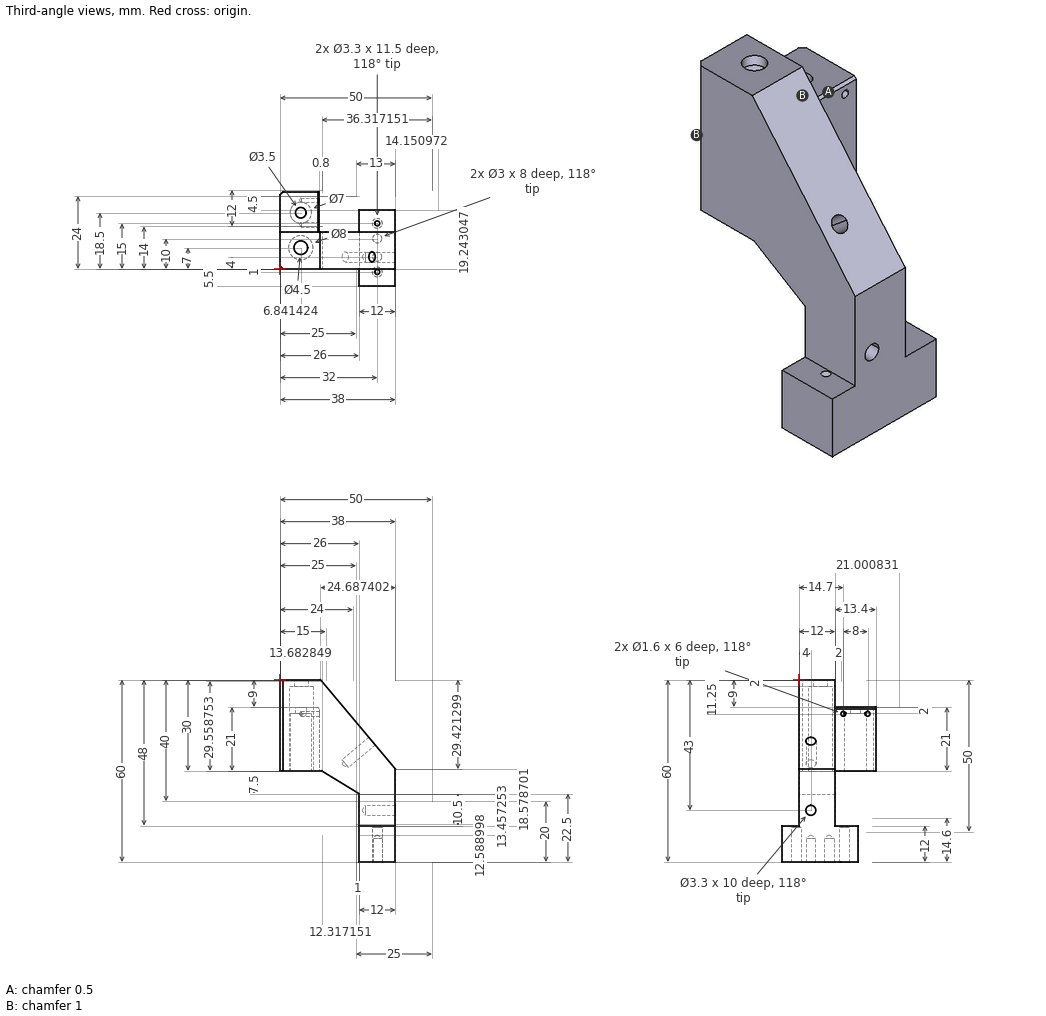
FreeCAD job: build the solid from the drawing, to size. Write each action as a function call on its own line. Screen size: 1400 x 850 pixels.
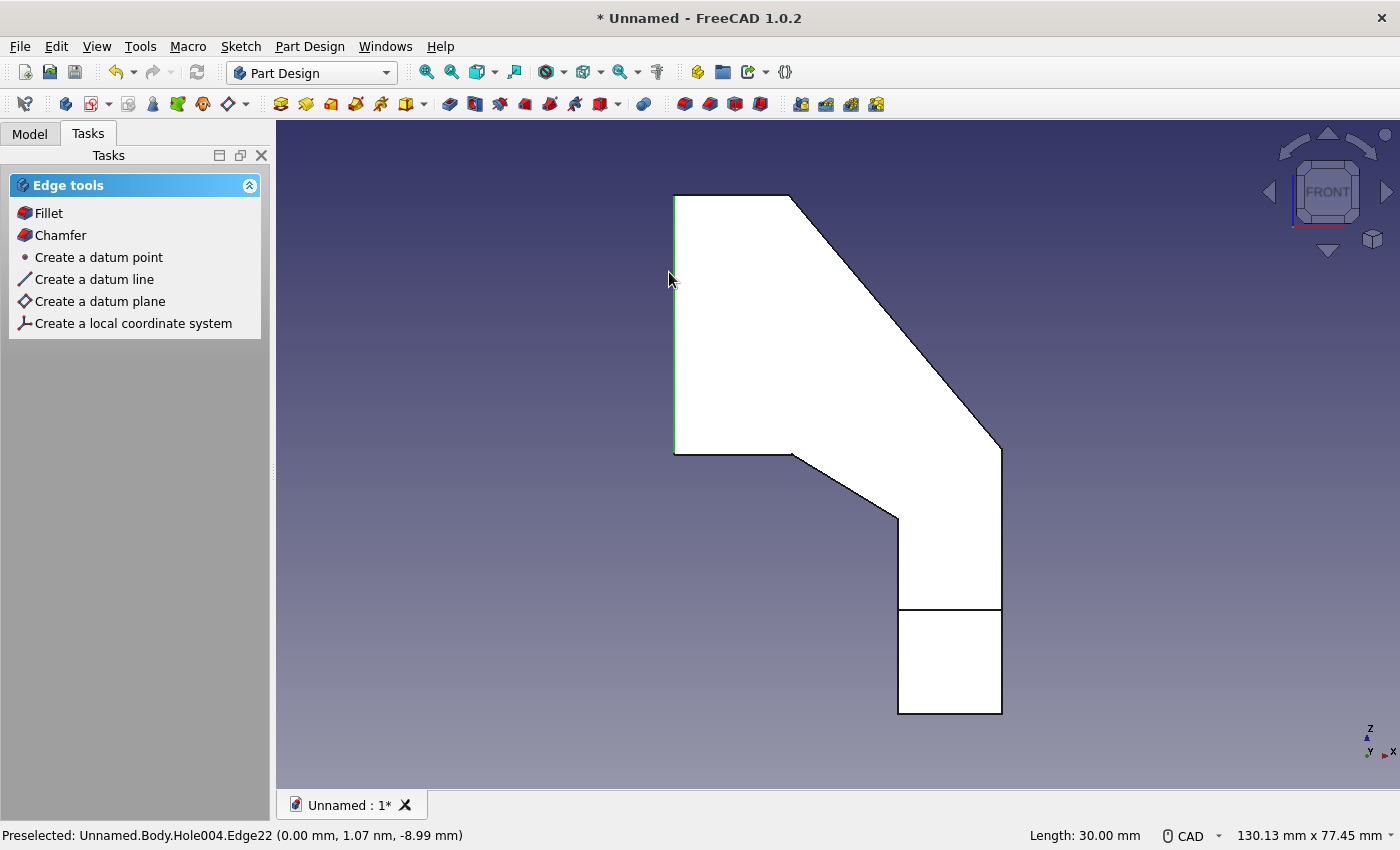
key(3)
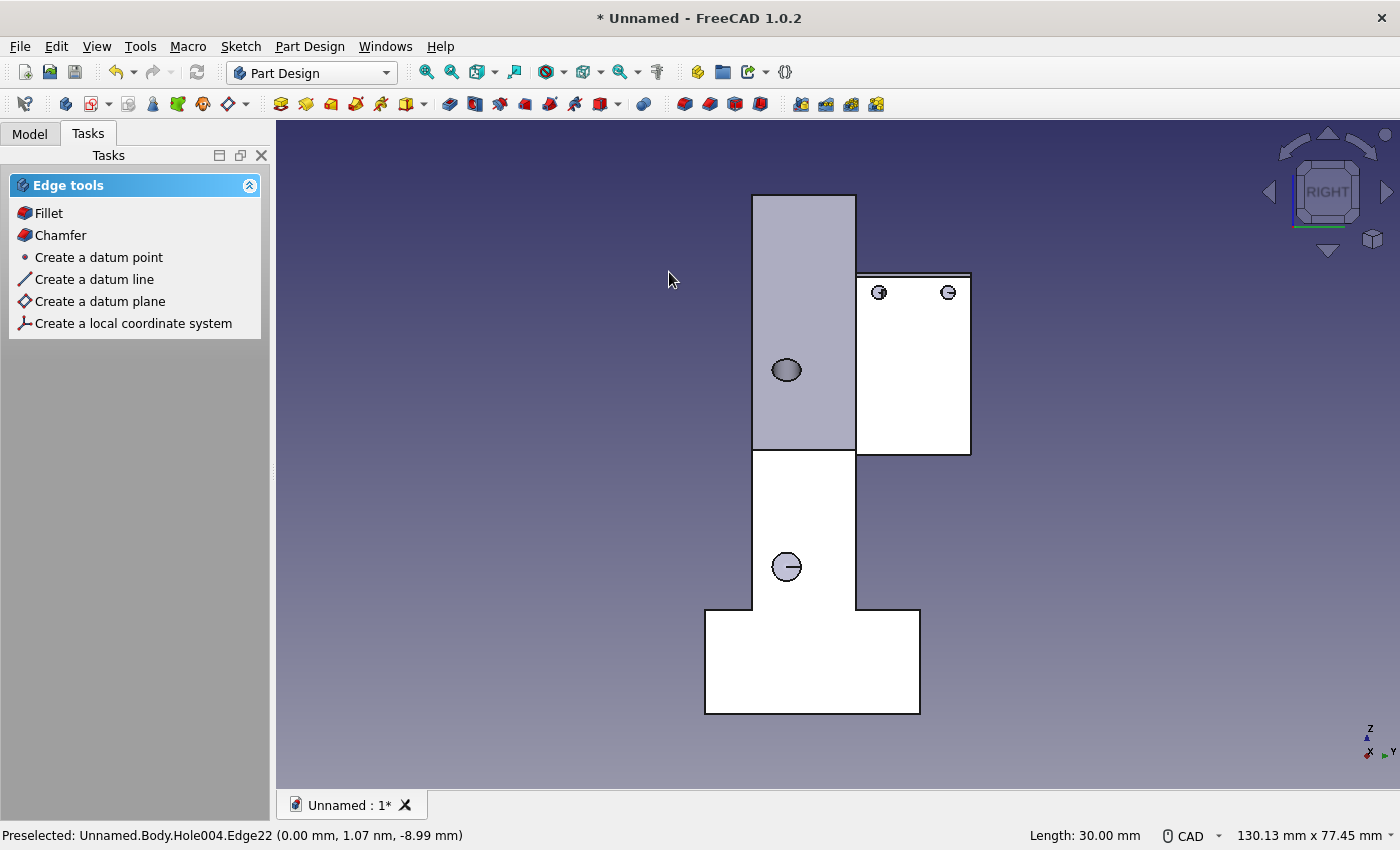
key(5)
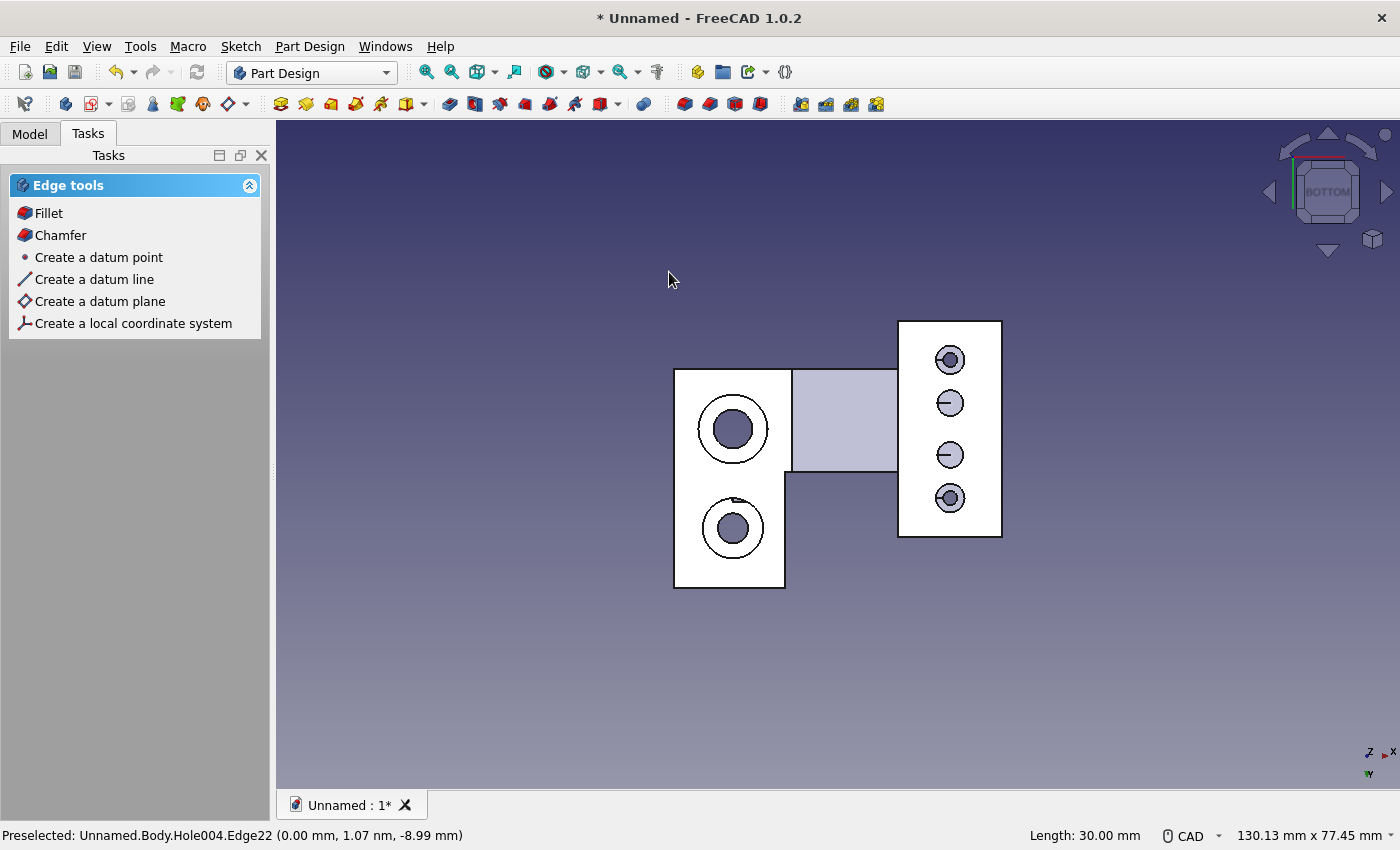
click(427, 72)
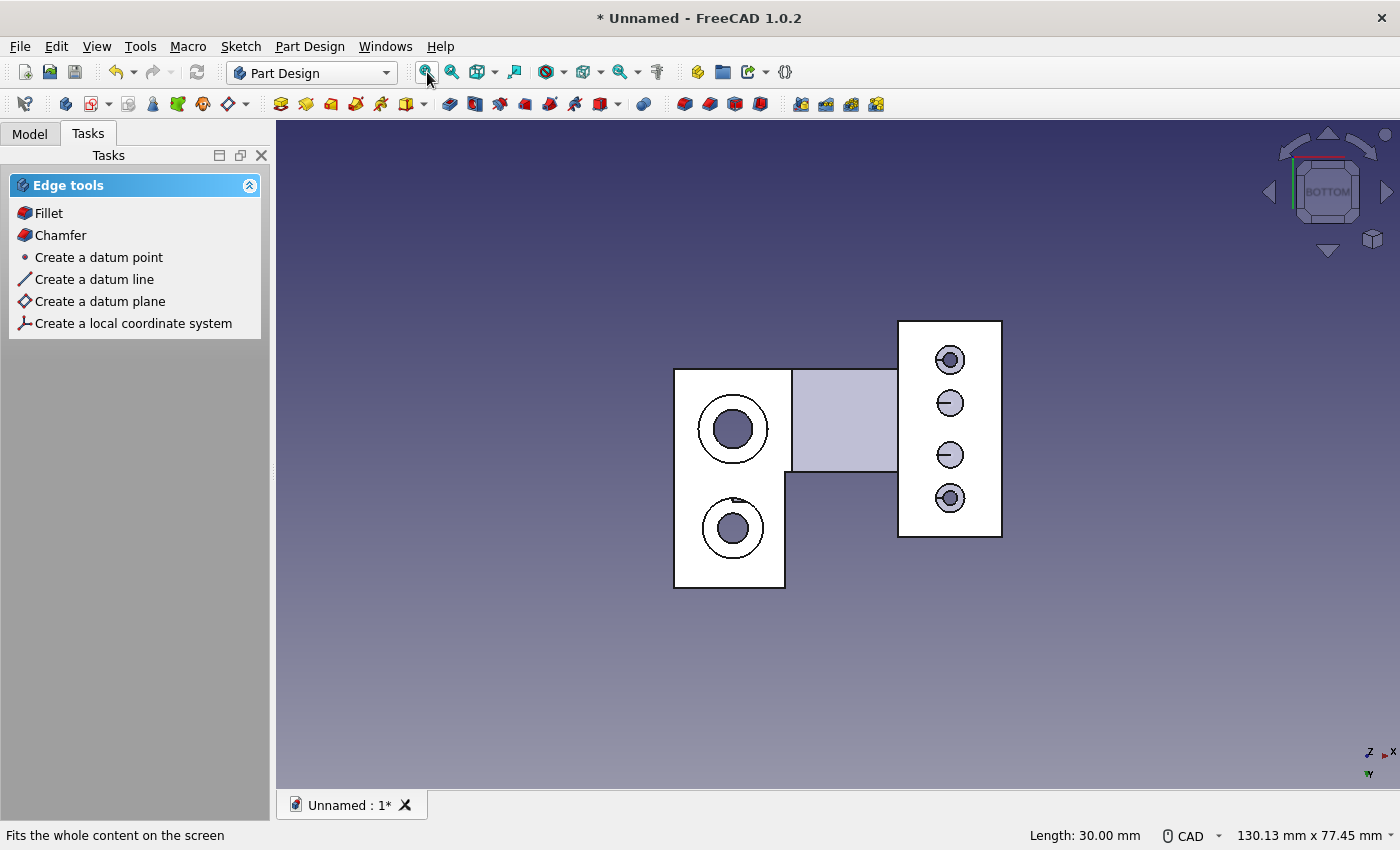
key(4)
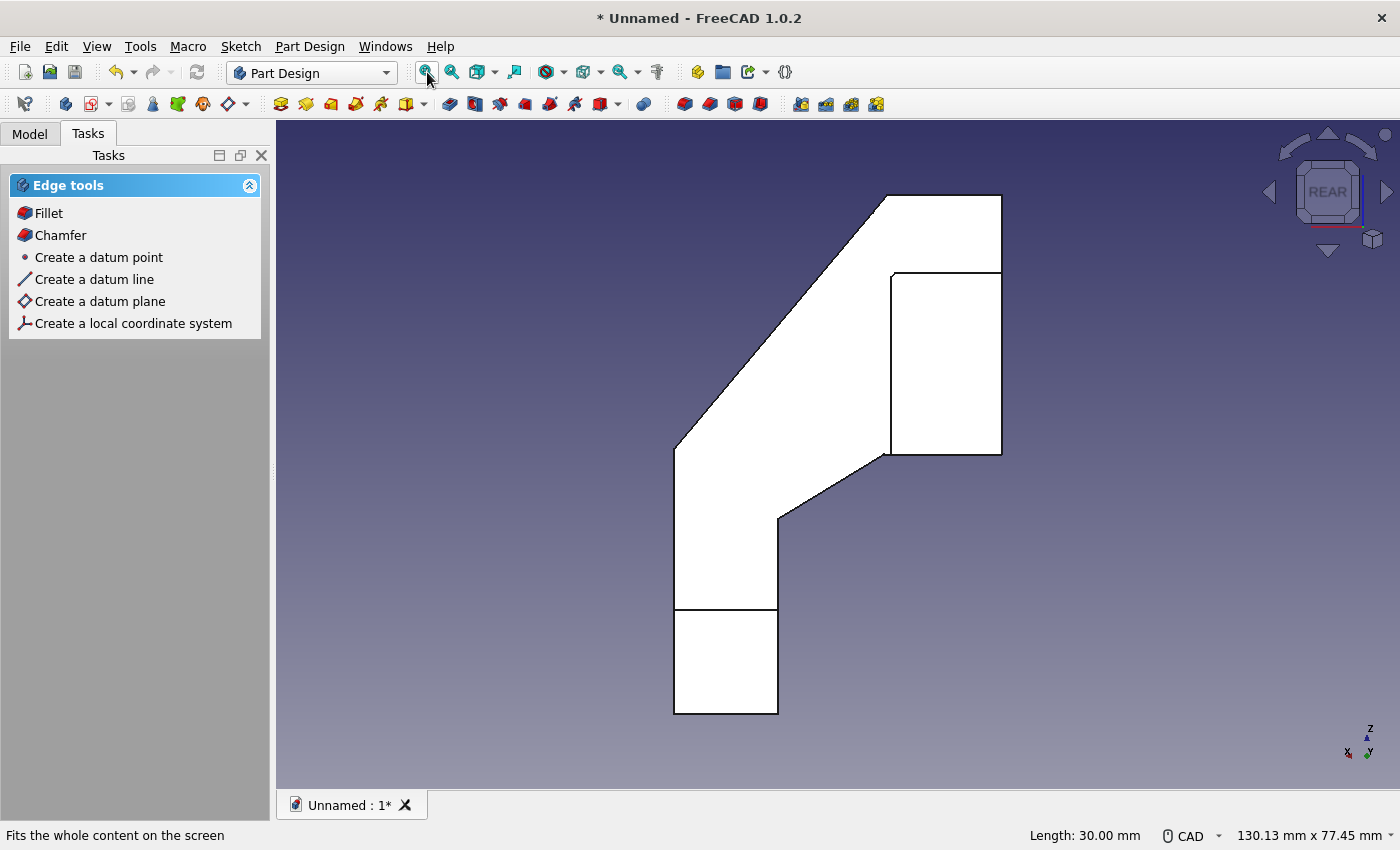
click(1002, 363, ctrl)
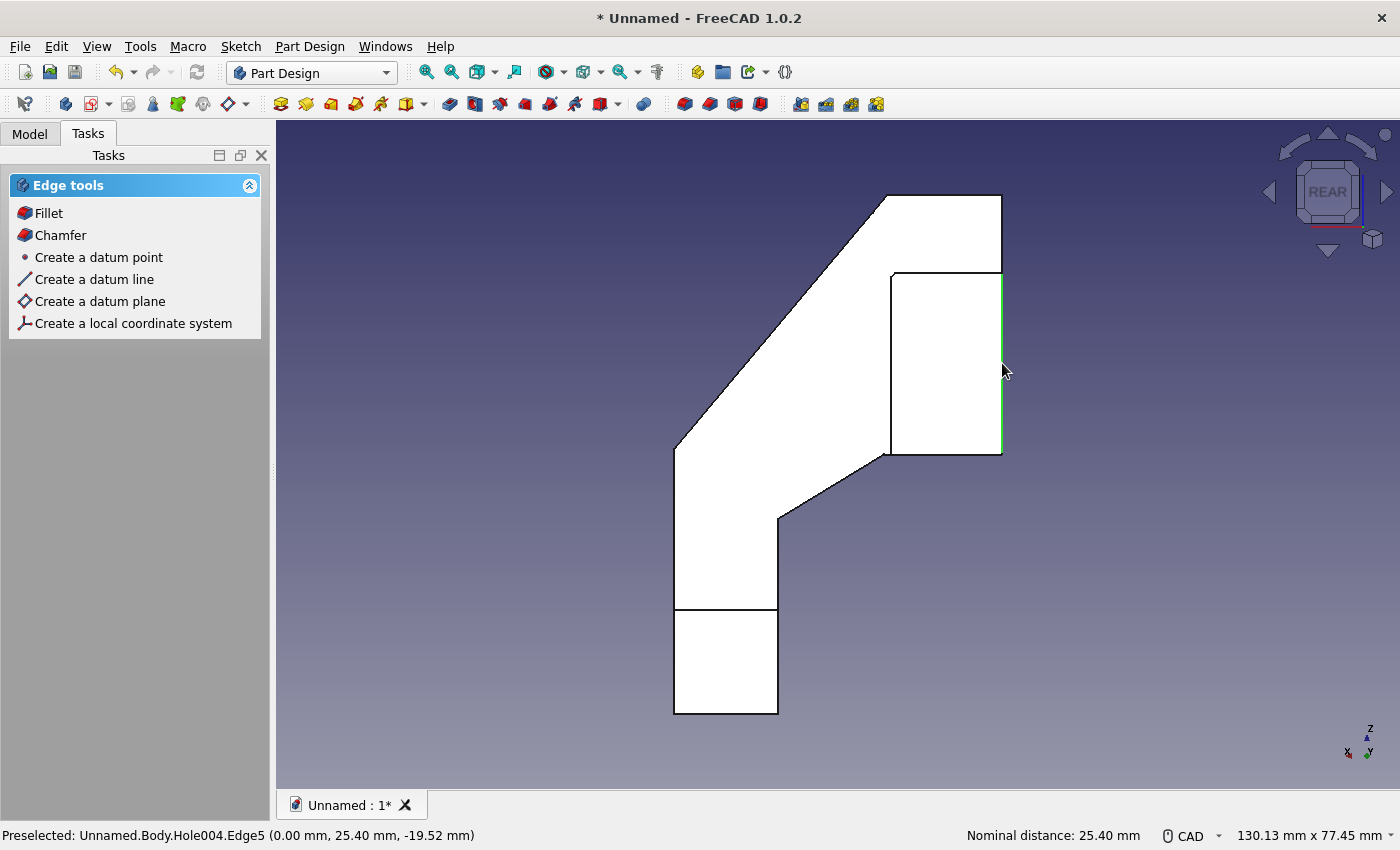
click(710, 104)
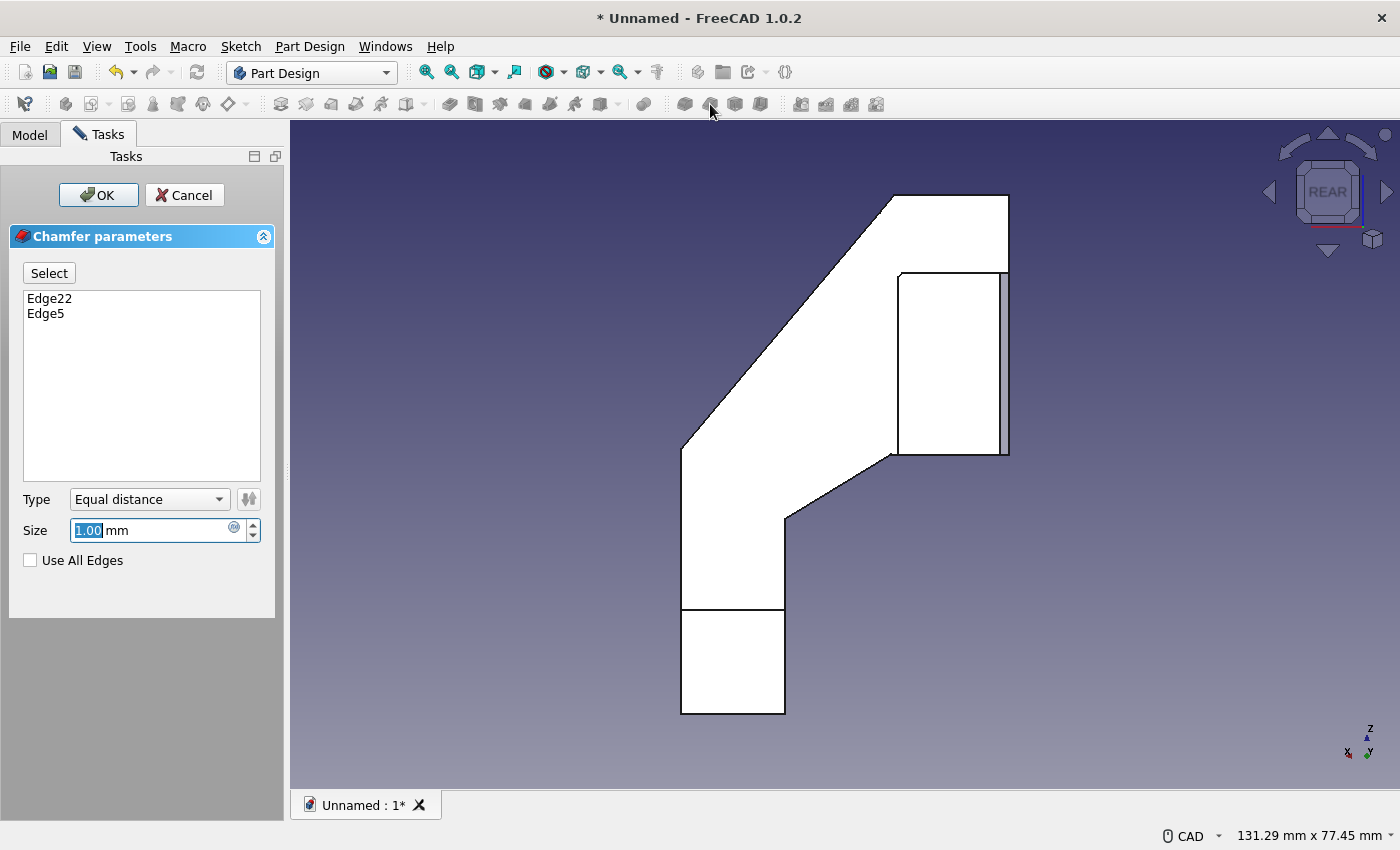
text(1)
key(Tab)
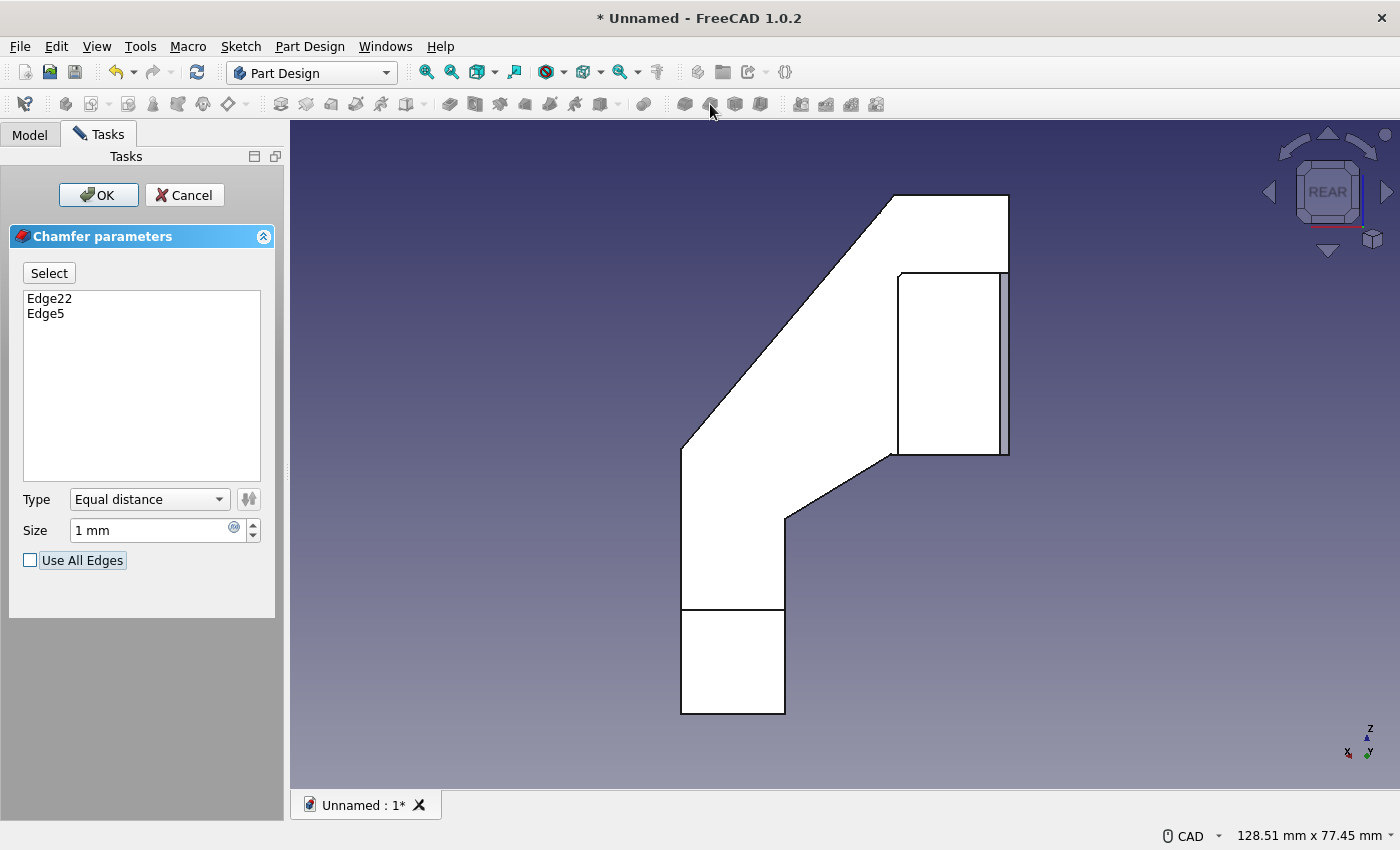
click(99, 195)